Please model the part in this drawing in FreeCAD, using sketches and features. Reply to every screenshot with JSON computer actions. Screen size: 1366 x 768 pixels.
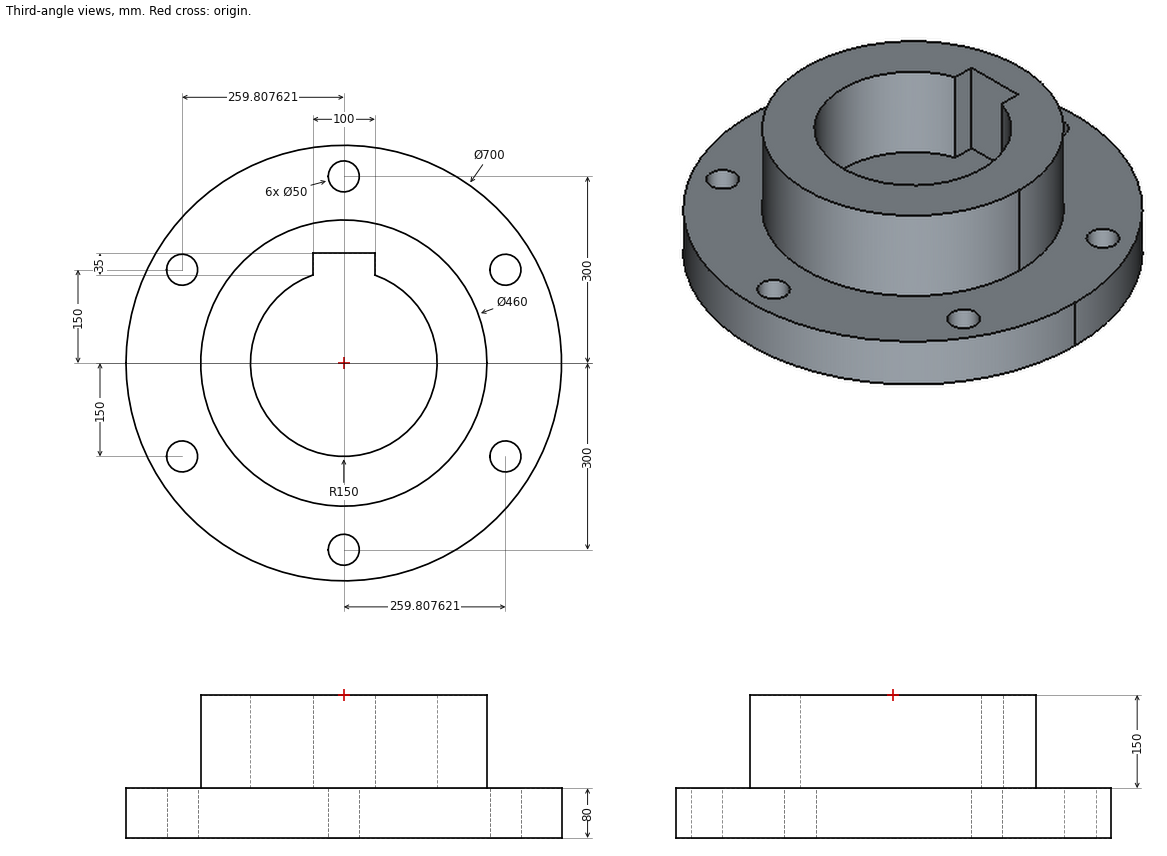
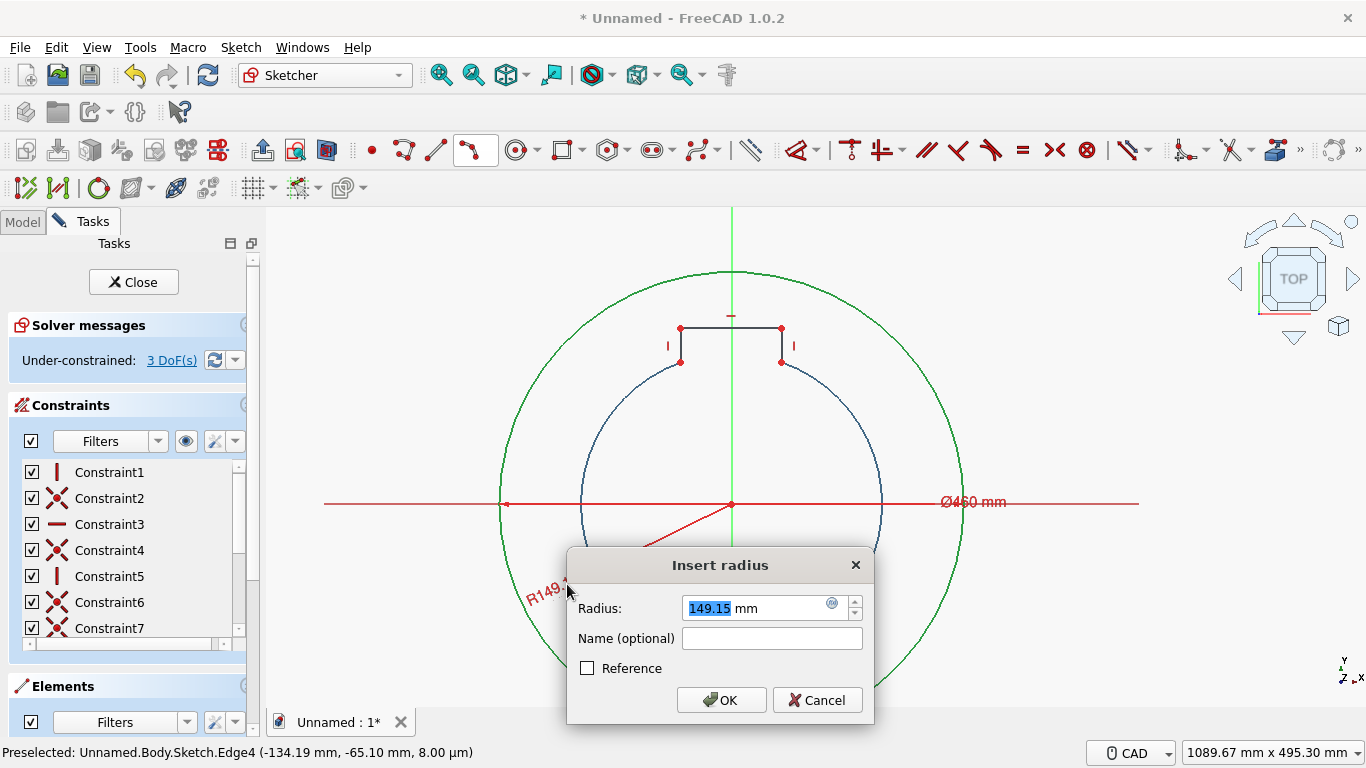
{"action": "type", "text": "150"}
{"action": "key", "text": "Return"}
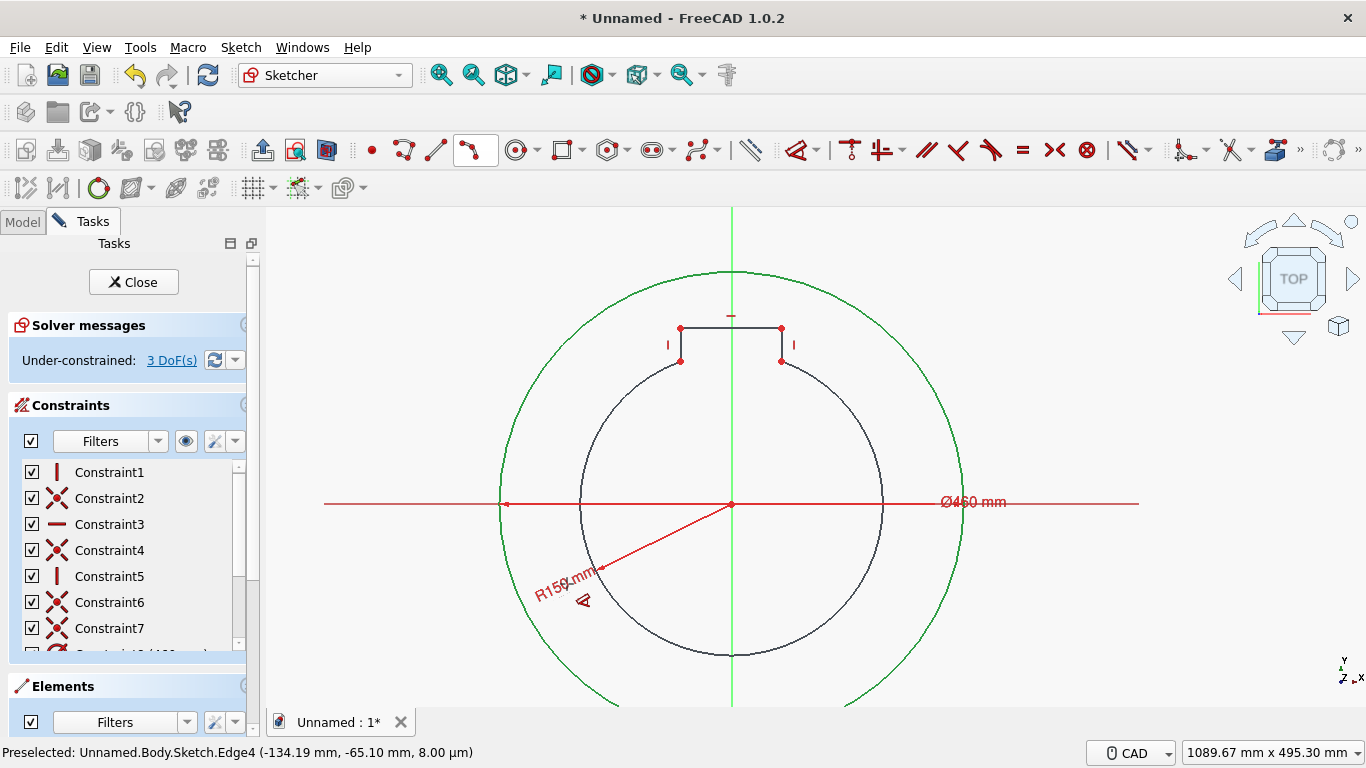
{"action": "scroll", "coordinate": [681, 352], "scroll_direction": "up", "scroll_amount": 2}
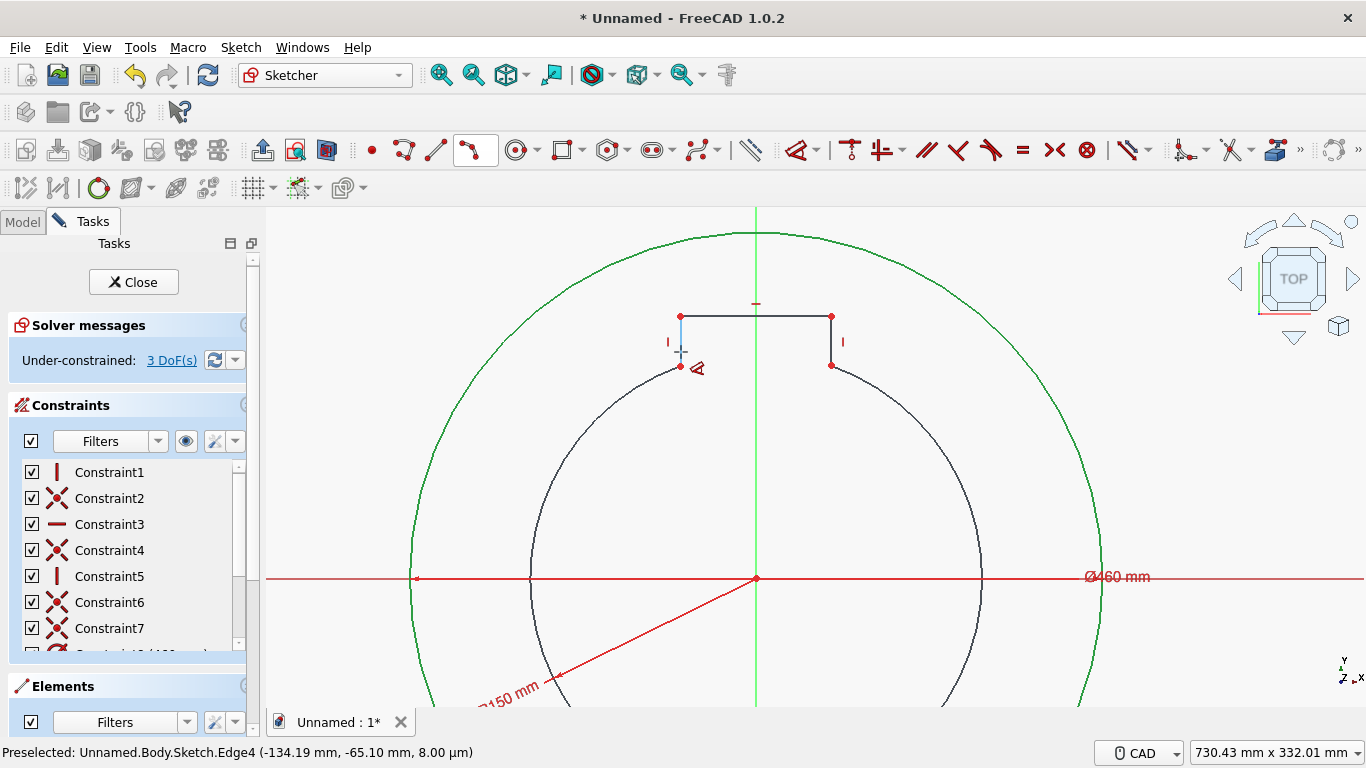
{"action": "left_click", "coordinate": [681, 351]}
{"action": "left_click", "coordinate": [647, 341]}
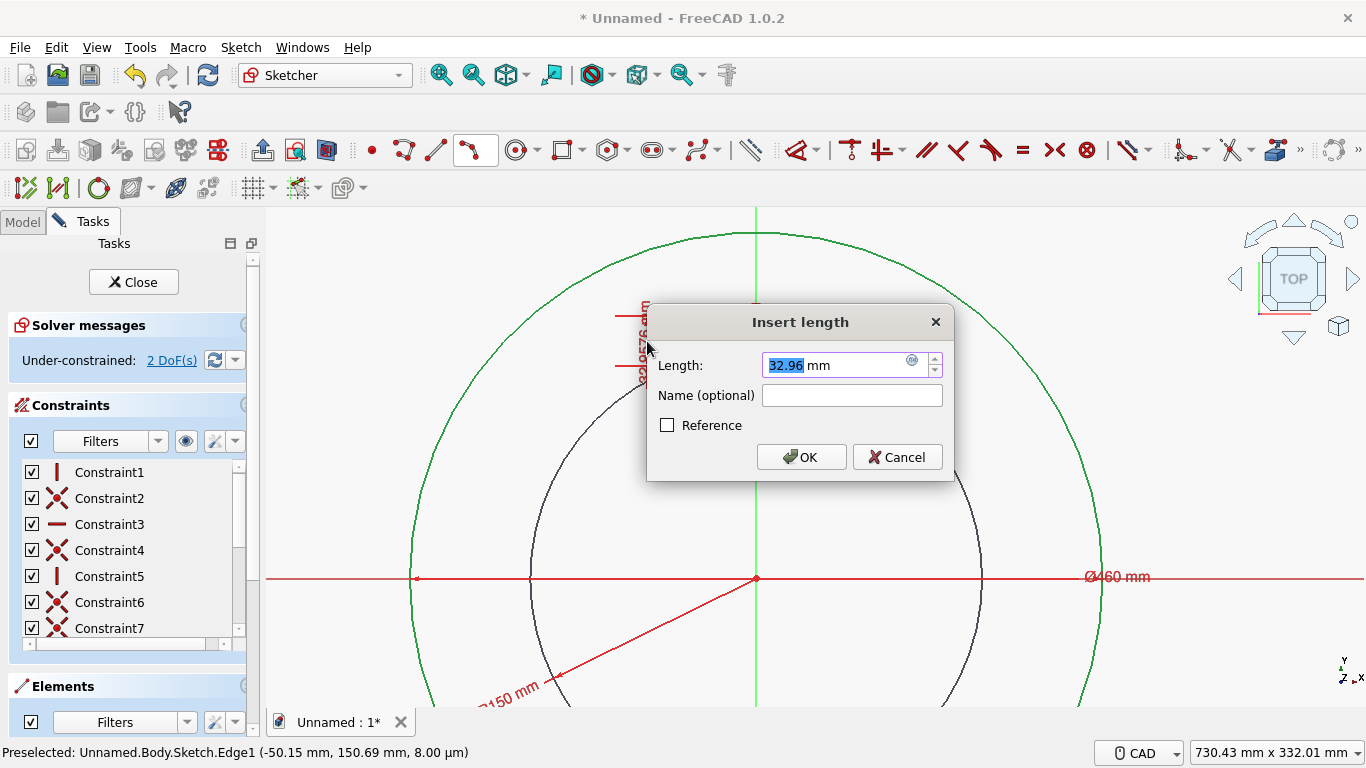
{"action": "type", "text": "35"}
{"action": "key", "text": "Return"}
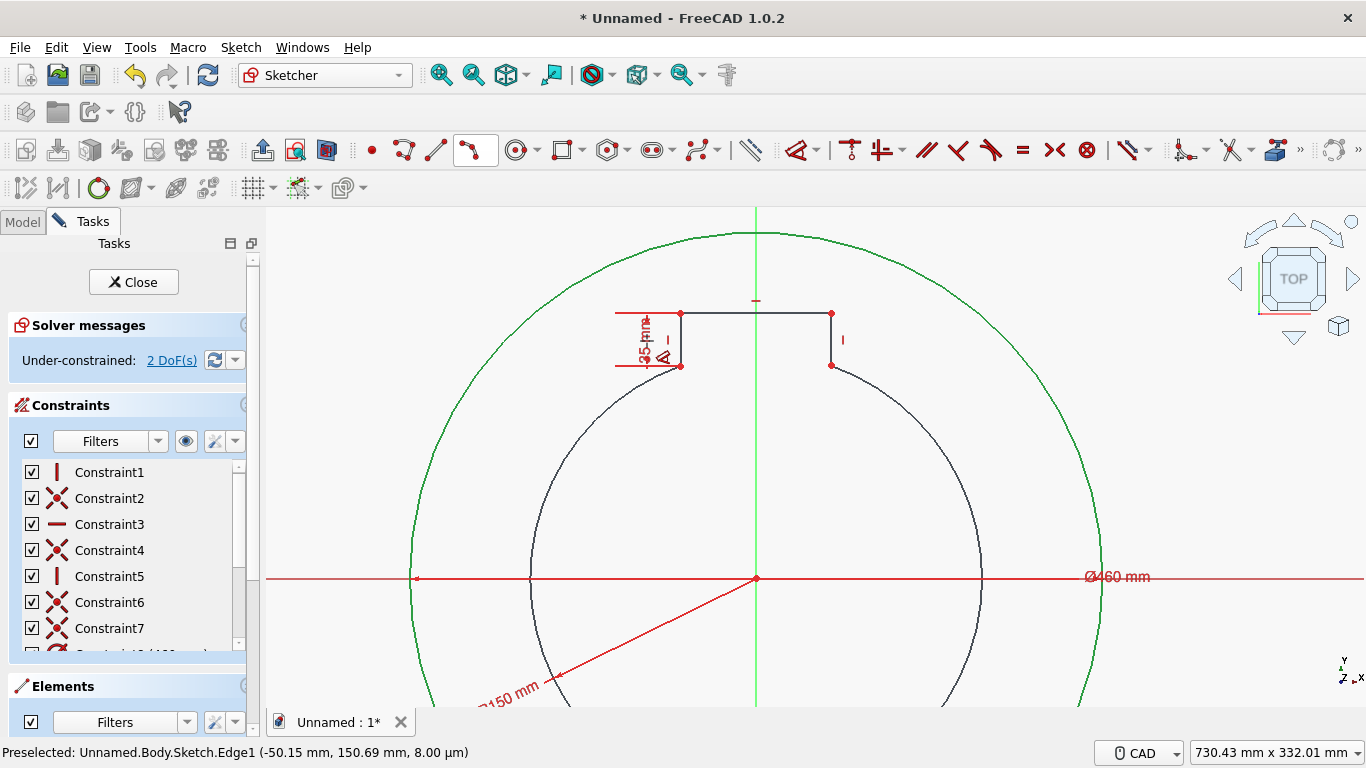
{"action": "left_click", "coordinate": [831, 329]}
{"action": "left_click", "coordinate": [865, 340]}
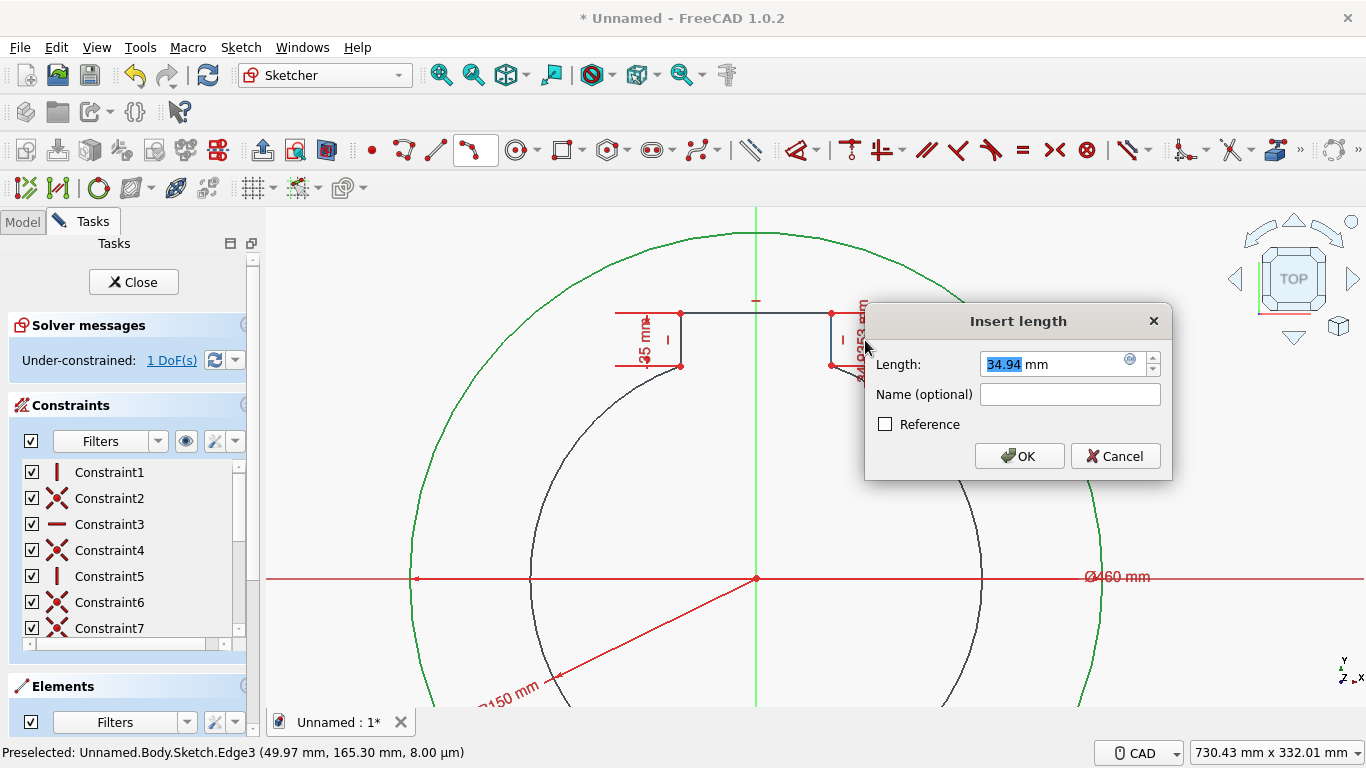
{"action": "type", "text": "35"}
{"action": "key", "text": "Return"}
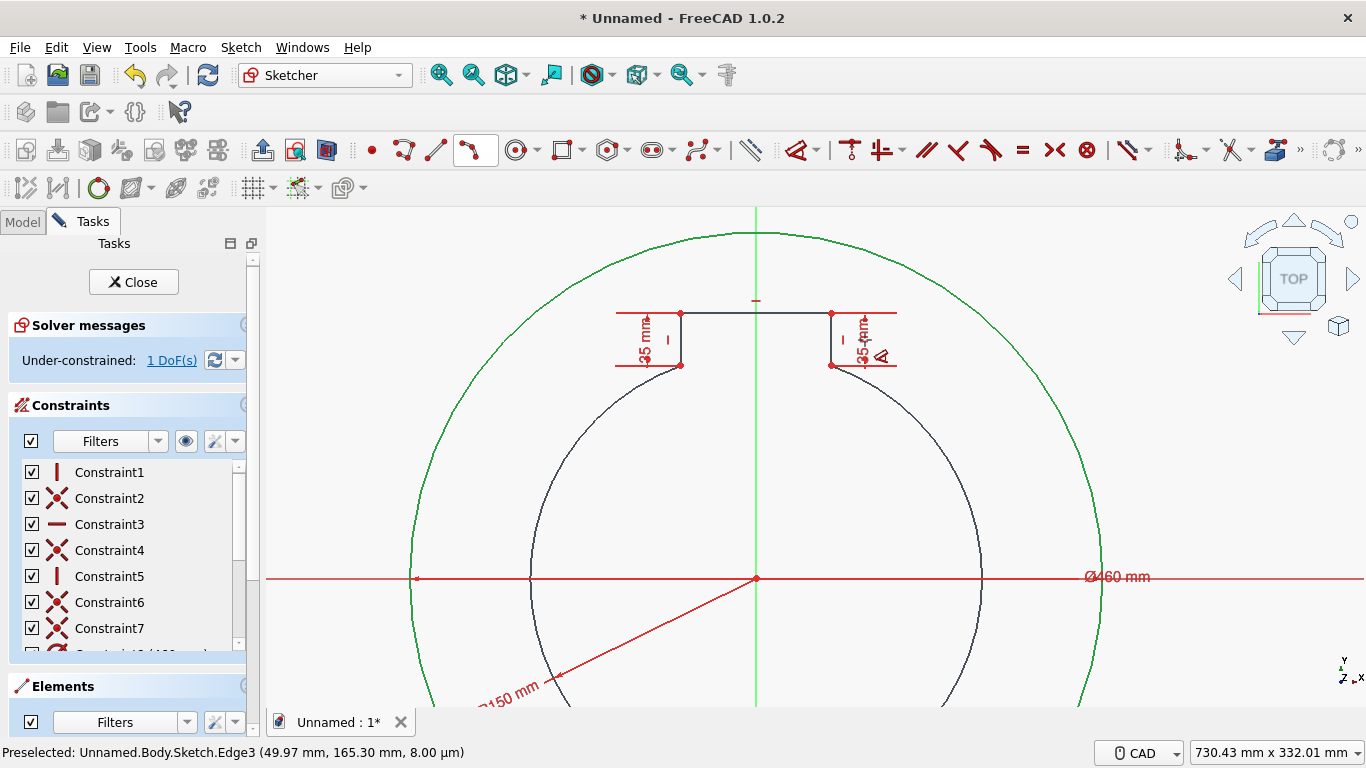
{"action": "left_click", "coordinate": [726, 313]}
{"action": "left_click", "coordinate": [722, 279]}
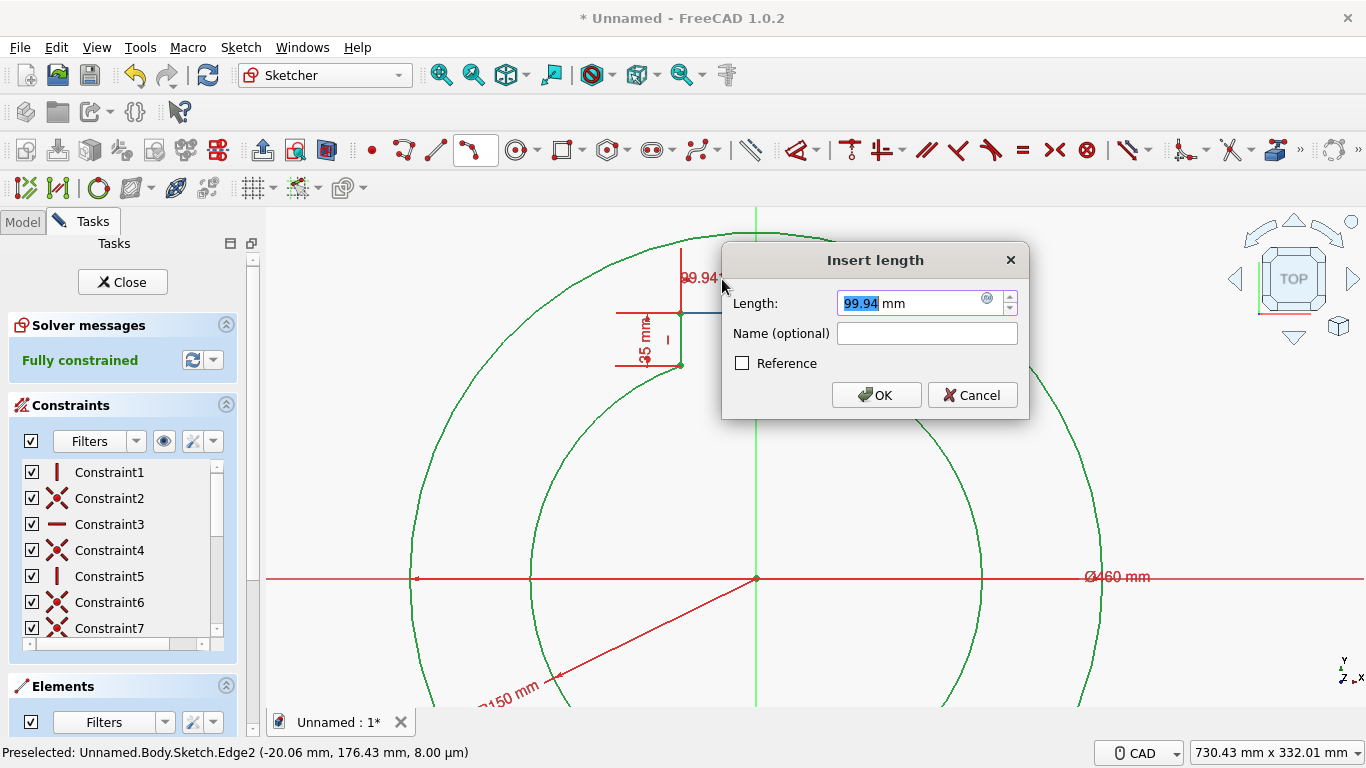
{"action": "type", "text": "100"}
{"action": "key", "text": "Return"}
{"action": "key", "text": "Escape"}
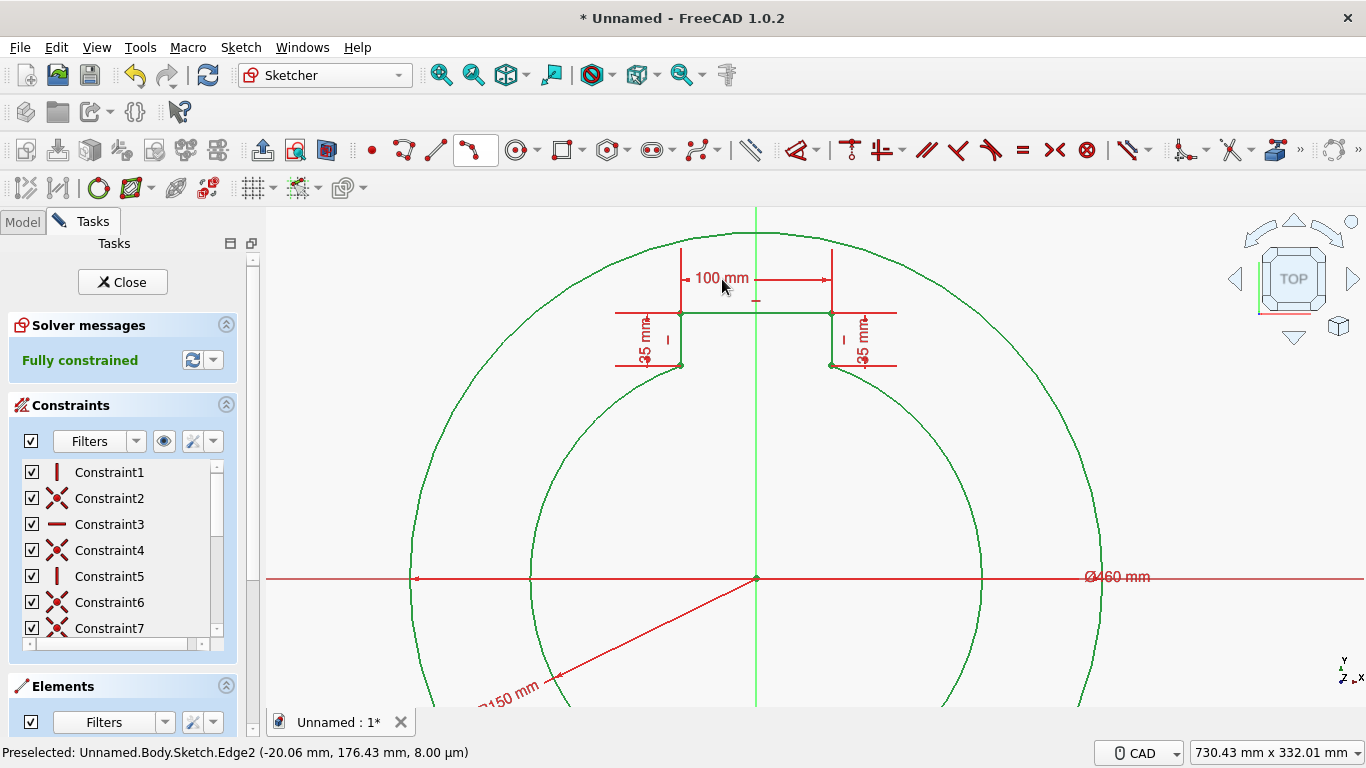
{"action": "left_click", "coordinate": [123, 282]}